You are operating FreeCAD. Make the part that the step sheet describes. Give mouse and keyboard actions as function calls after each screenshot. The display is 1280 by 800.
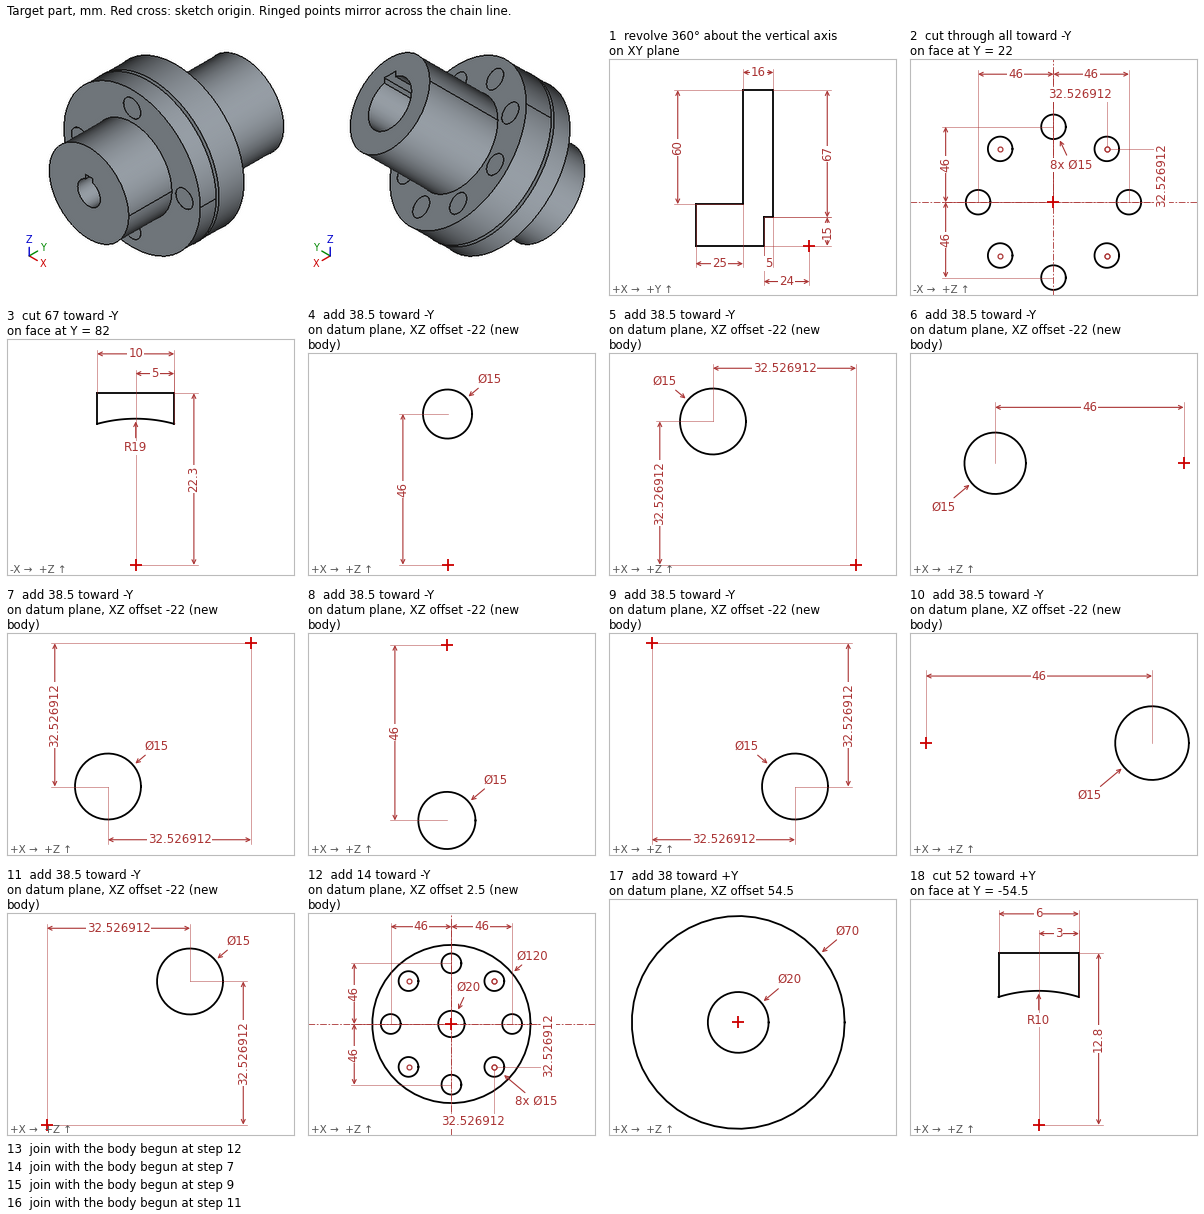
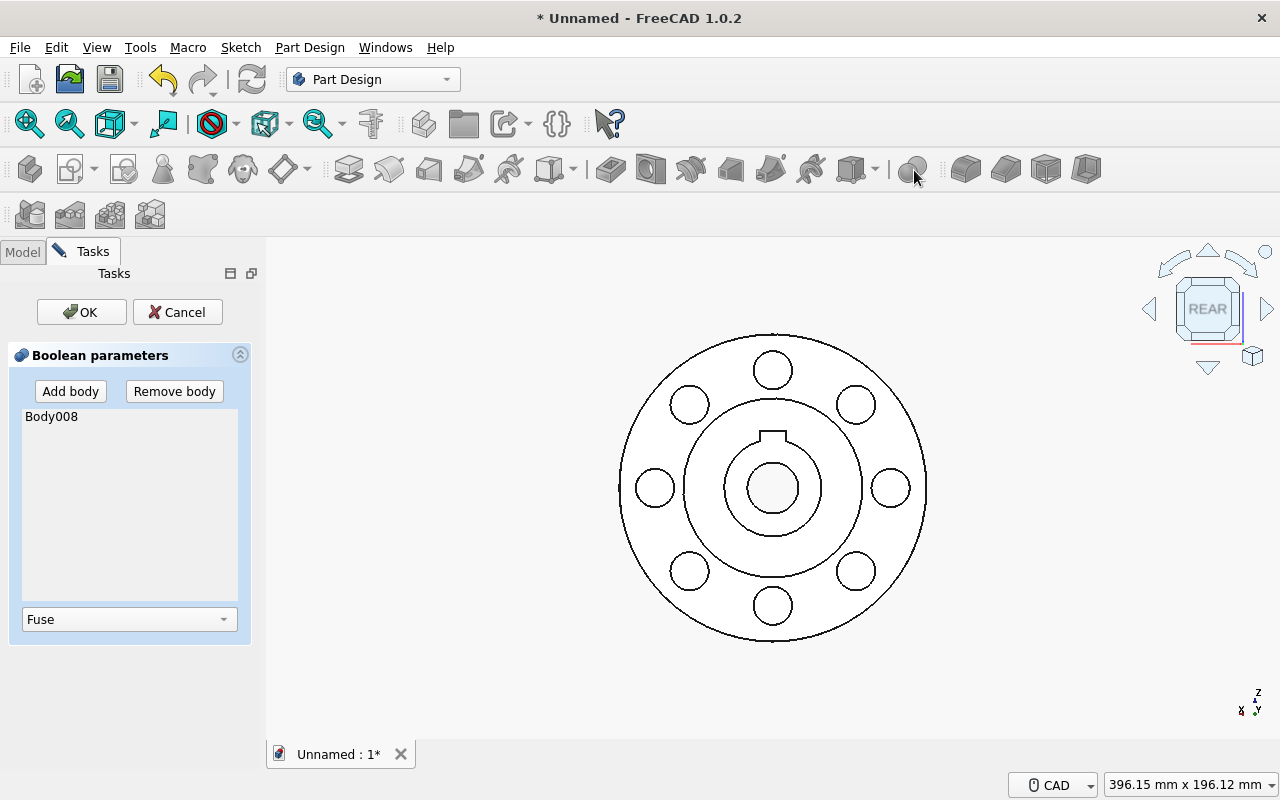
click(82, 312)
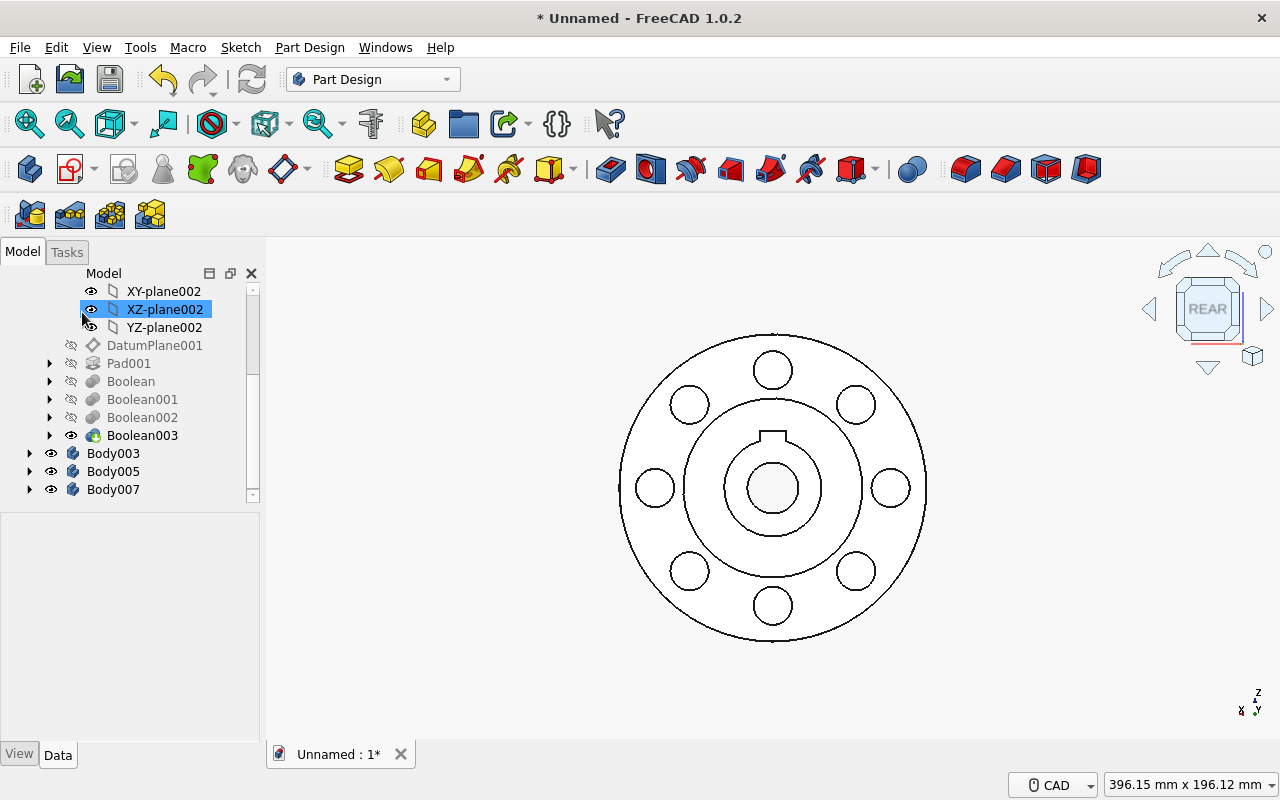
scroll(160, 395, down, 3)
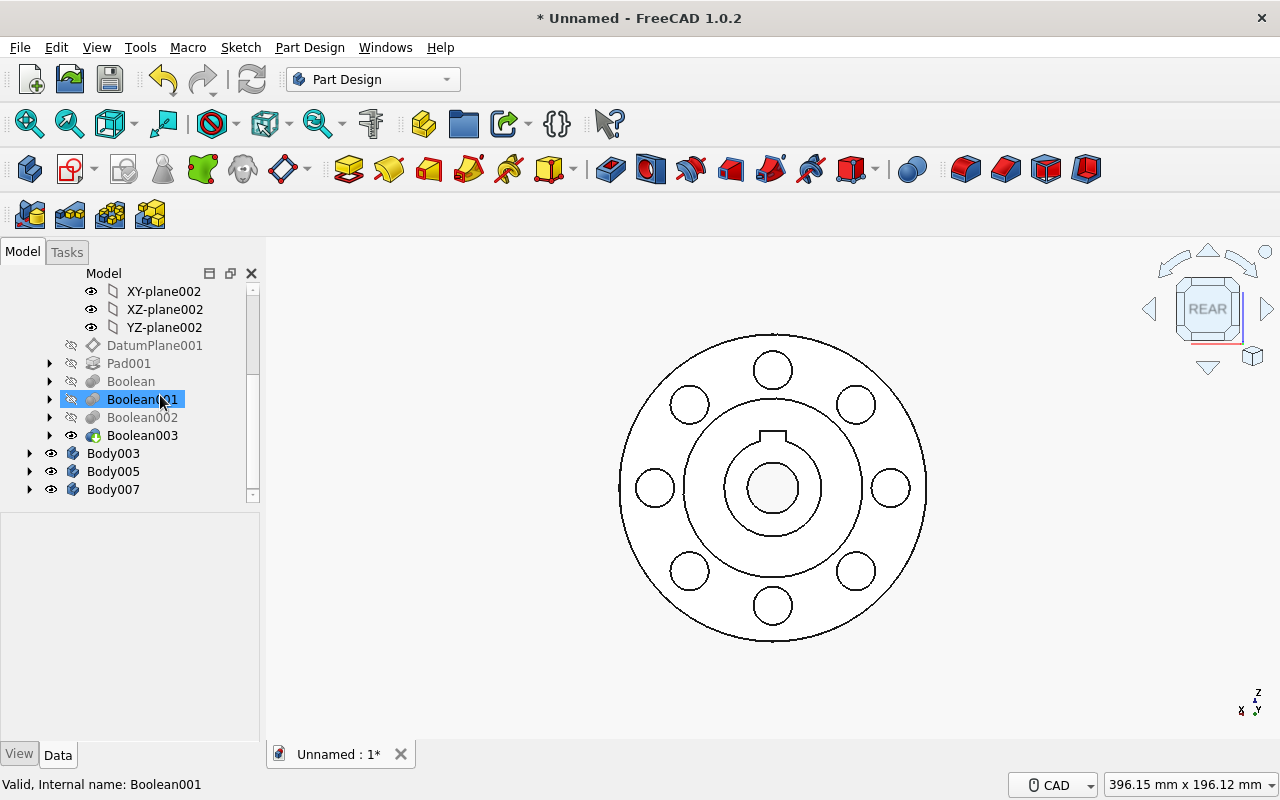
scroll(160, 395, up, 15)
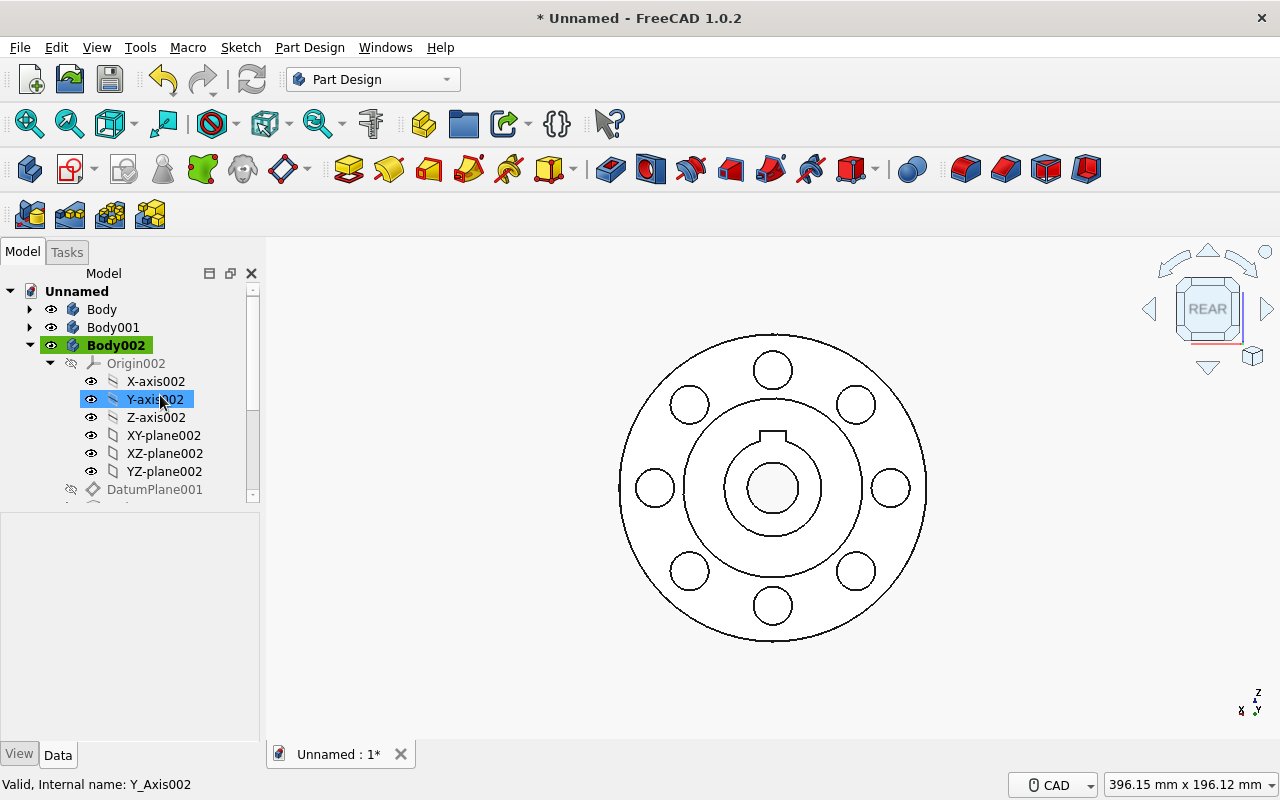
click(136, 453)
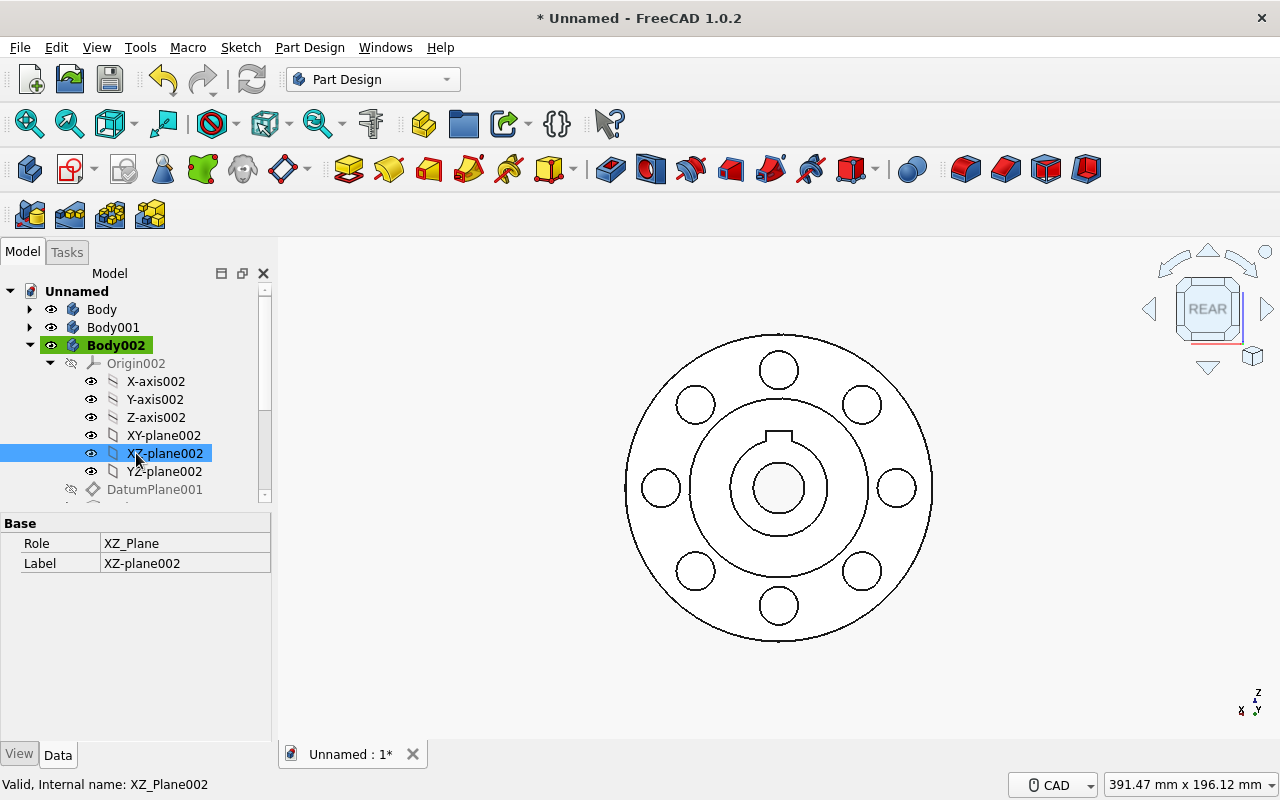
click(284, 170)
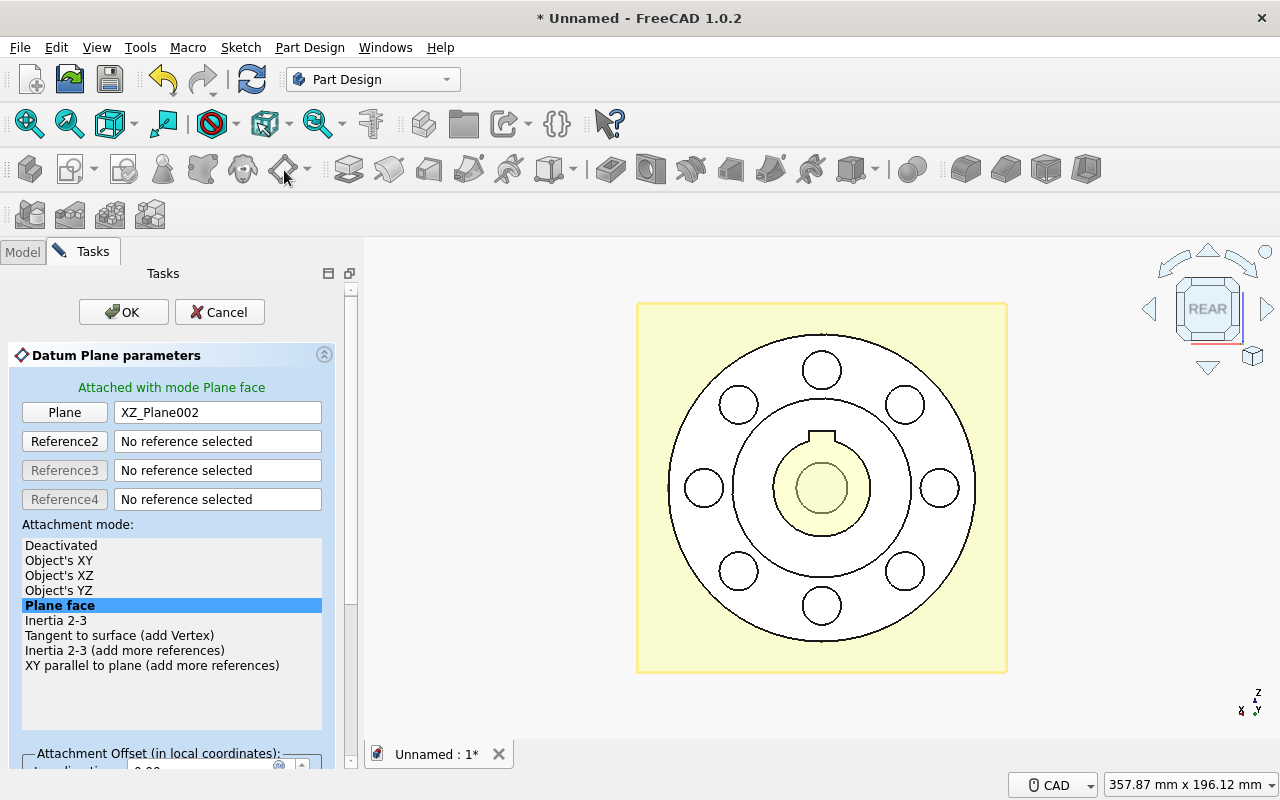
scroll(351, 526, down, 3)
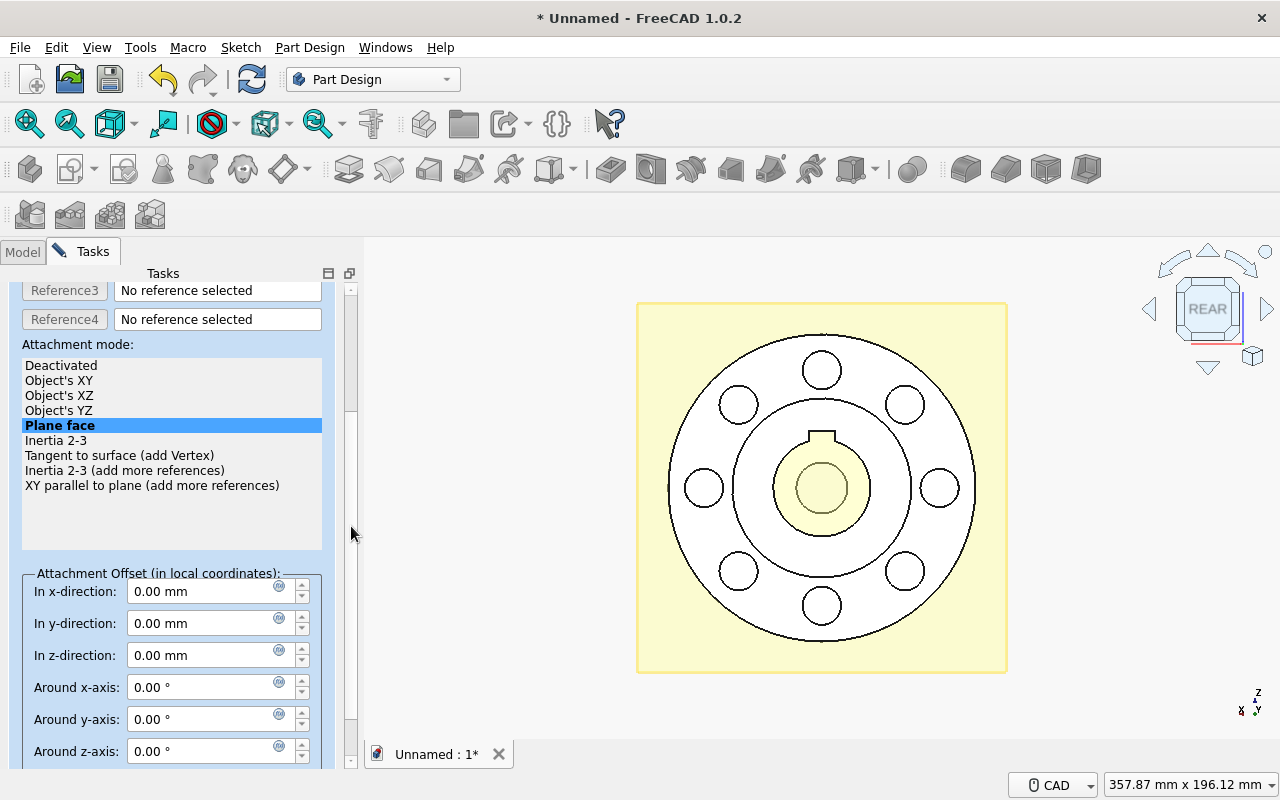
triple_click(210, 655)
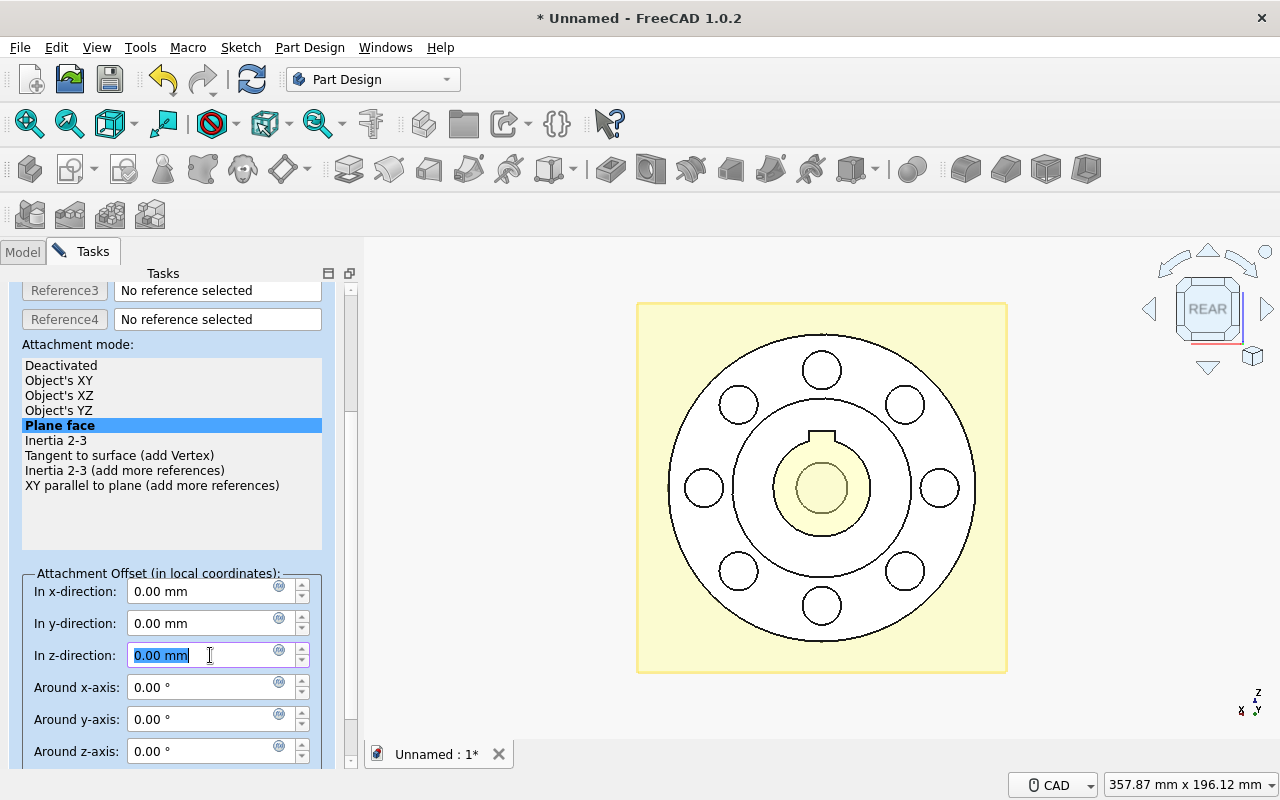
text(54.5)
key(Tab)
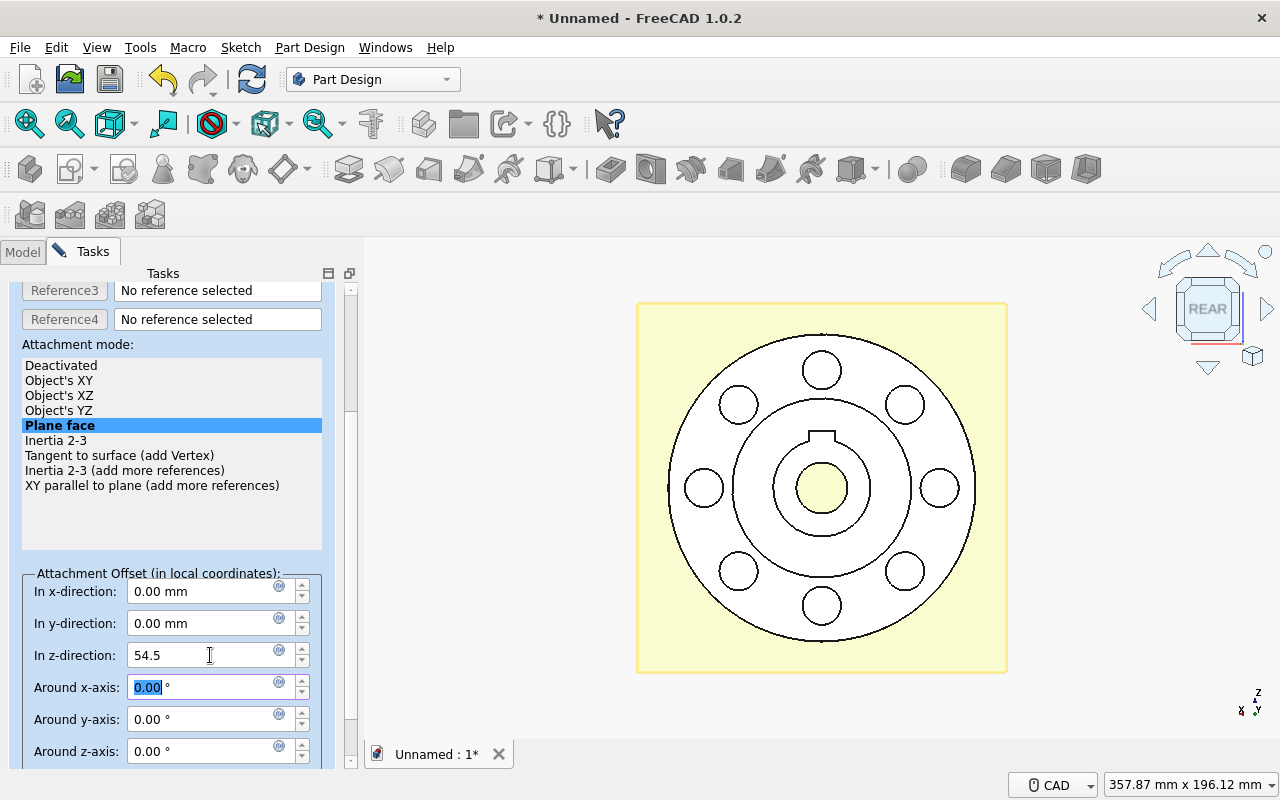
scroll(351, 526, up, 4)